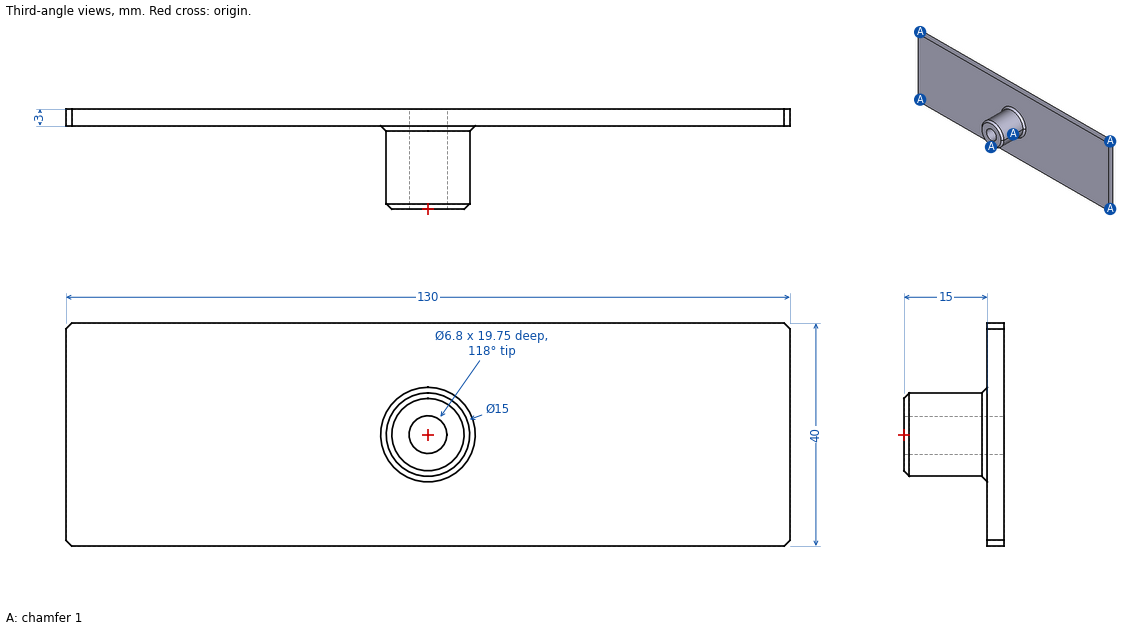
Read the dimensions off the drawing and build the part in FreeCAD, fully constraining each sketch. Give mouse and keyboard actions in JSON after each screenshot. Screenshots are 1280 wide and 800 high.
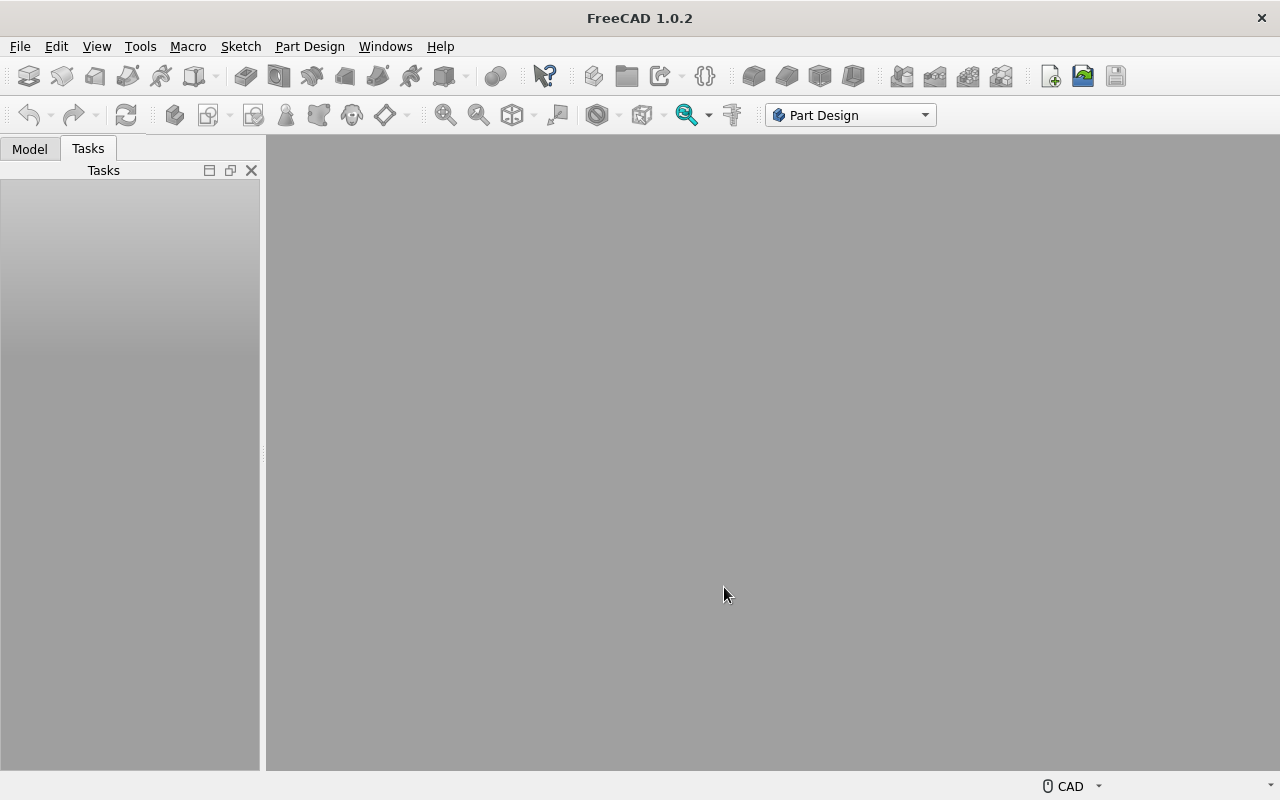
{"action": "left_click", "coordinate": [1050, 76]}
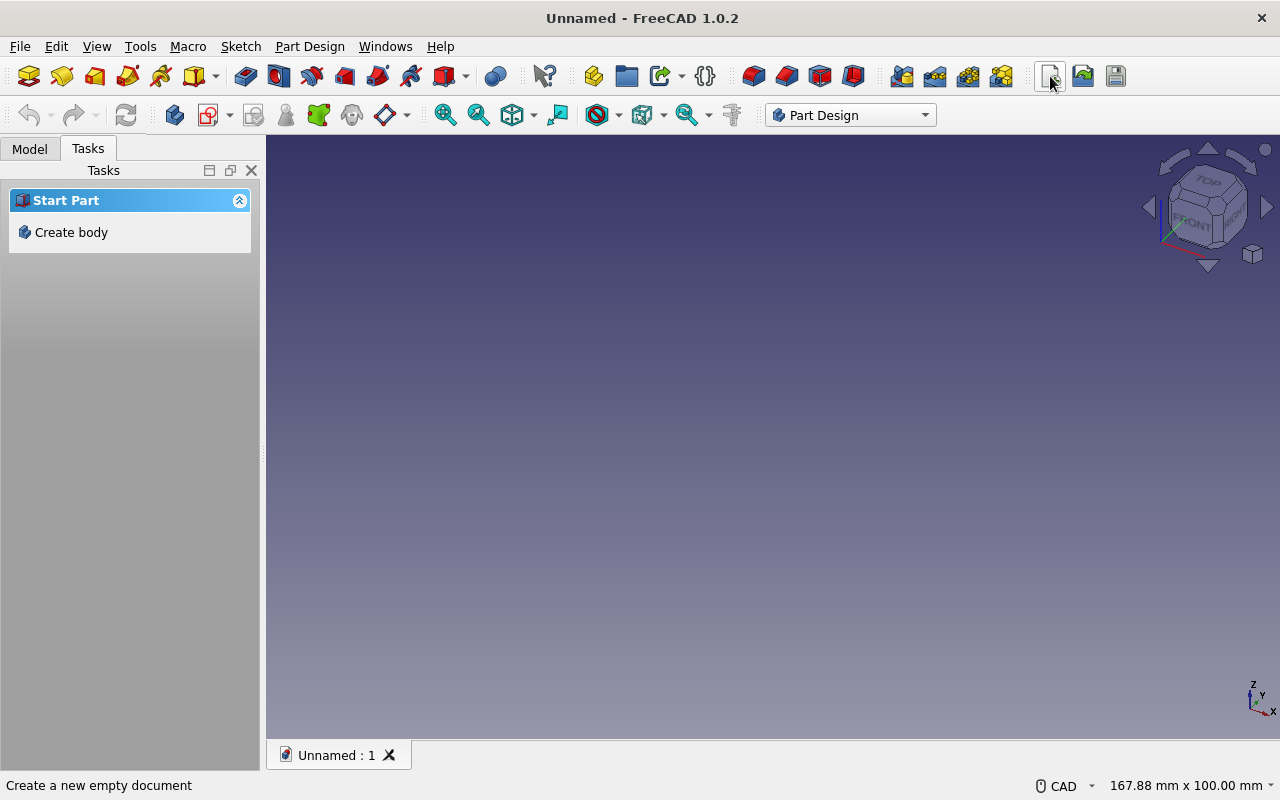
{"action": "left_click", "coordinate": [208, 116]}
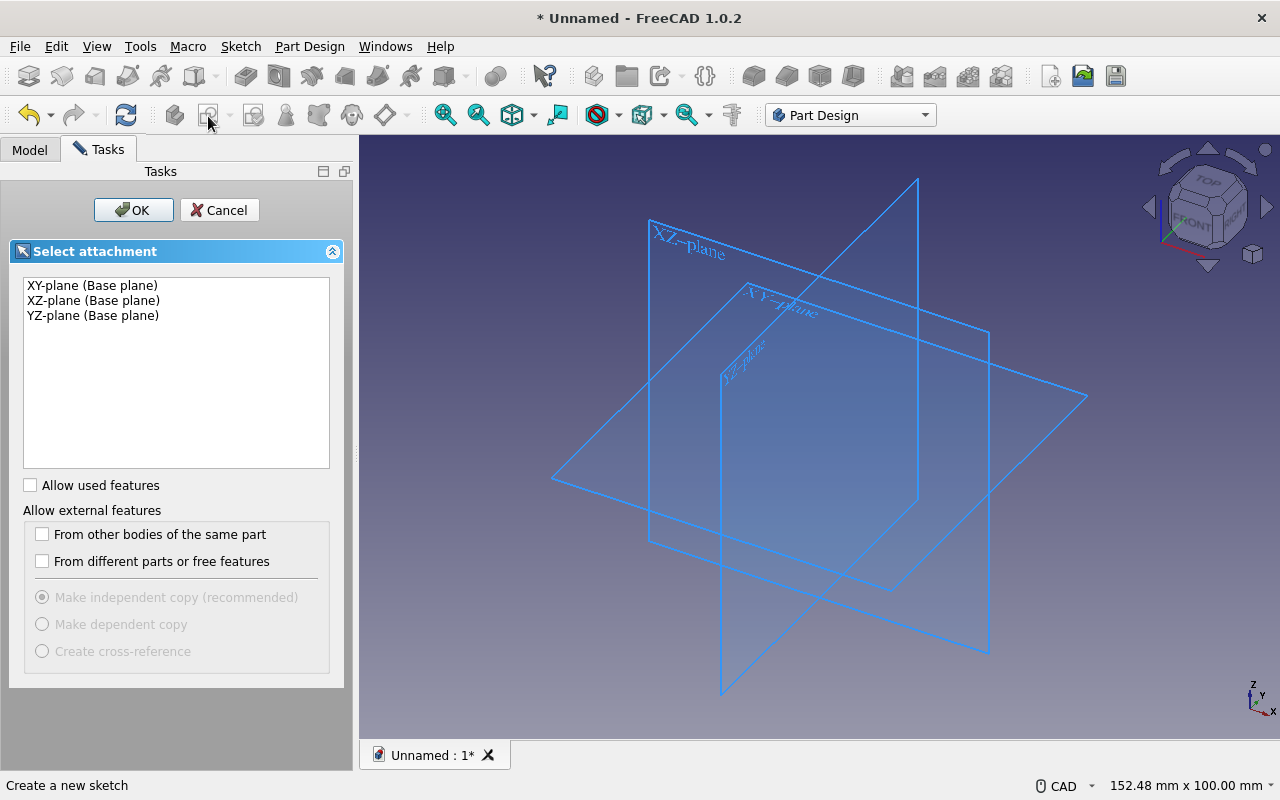
{"action": "left_click", "coordinate": [84, 300]}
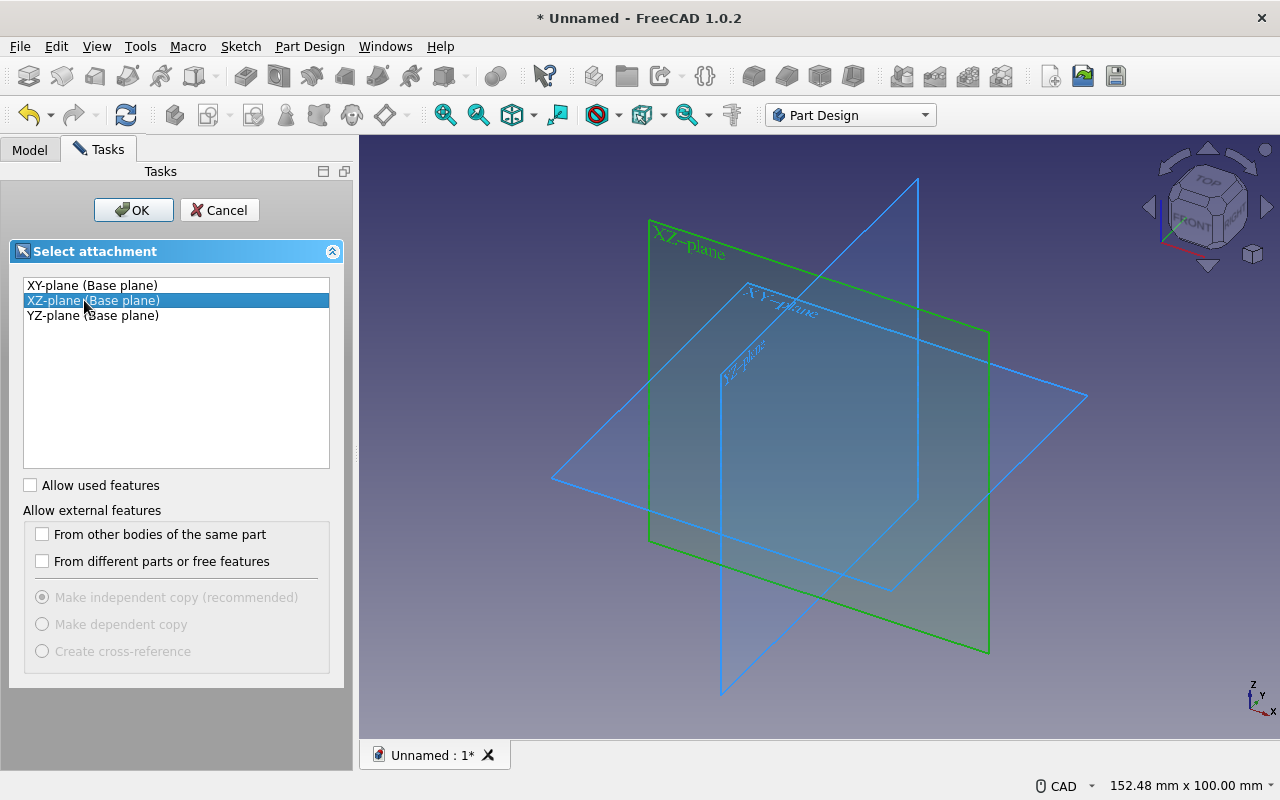
{"action": "left_click", "coordinate": [134, 210]}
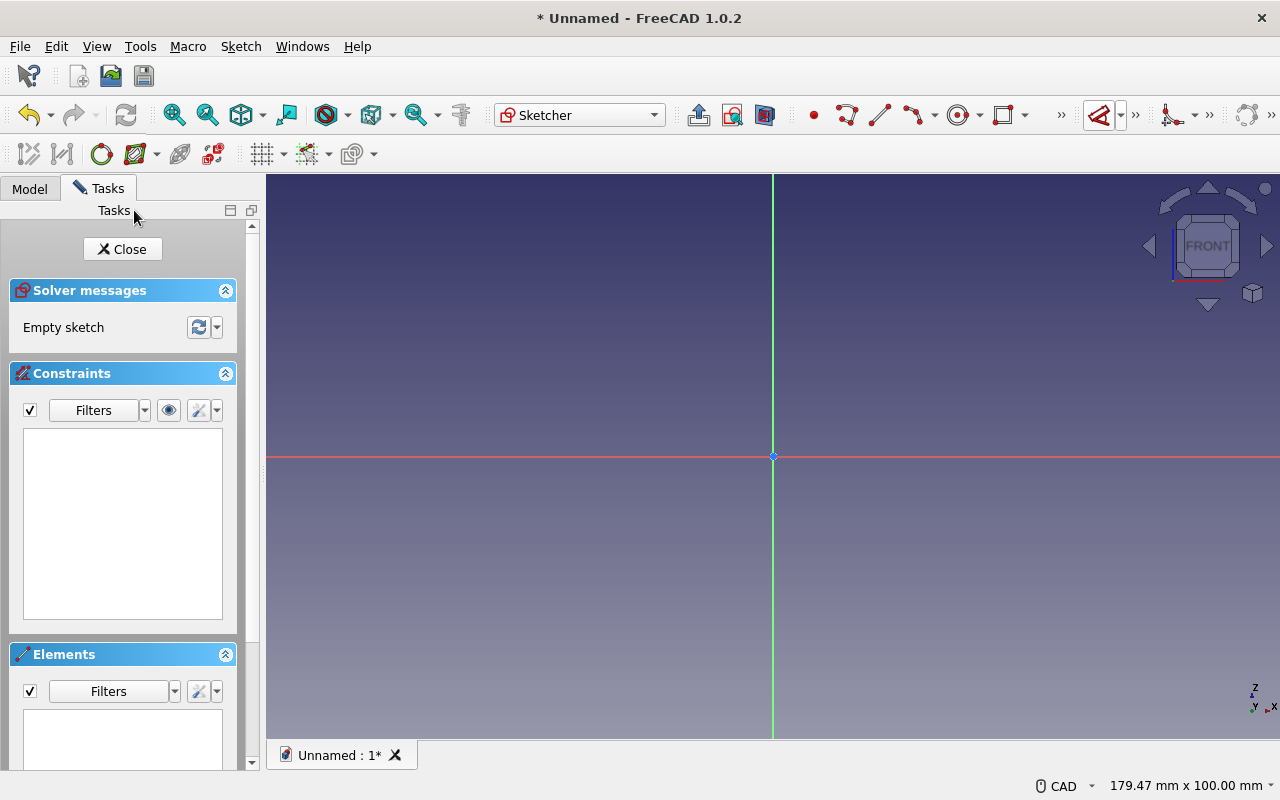
{"action": "scroll", "coordinate": [795, 456], "scroll_direction": "up", "scroll_amount": 7}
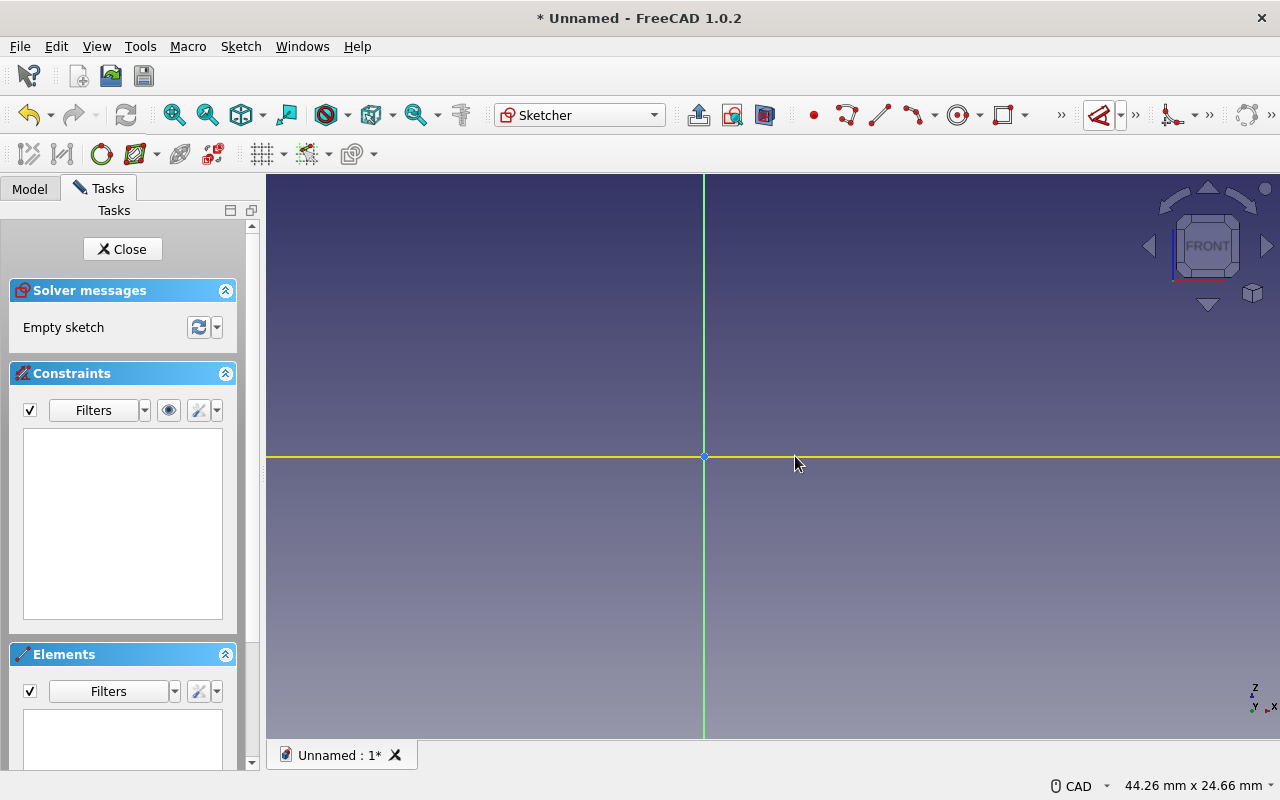
{"action": "left_click", "coordinate": [958, 116]}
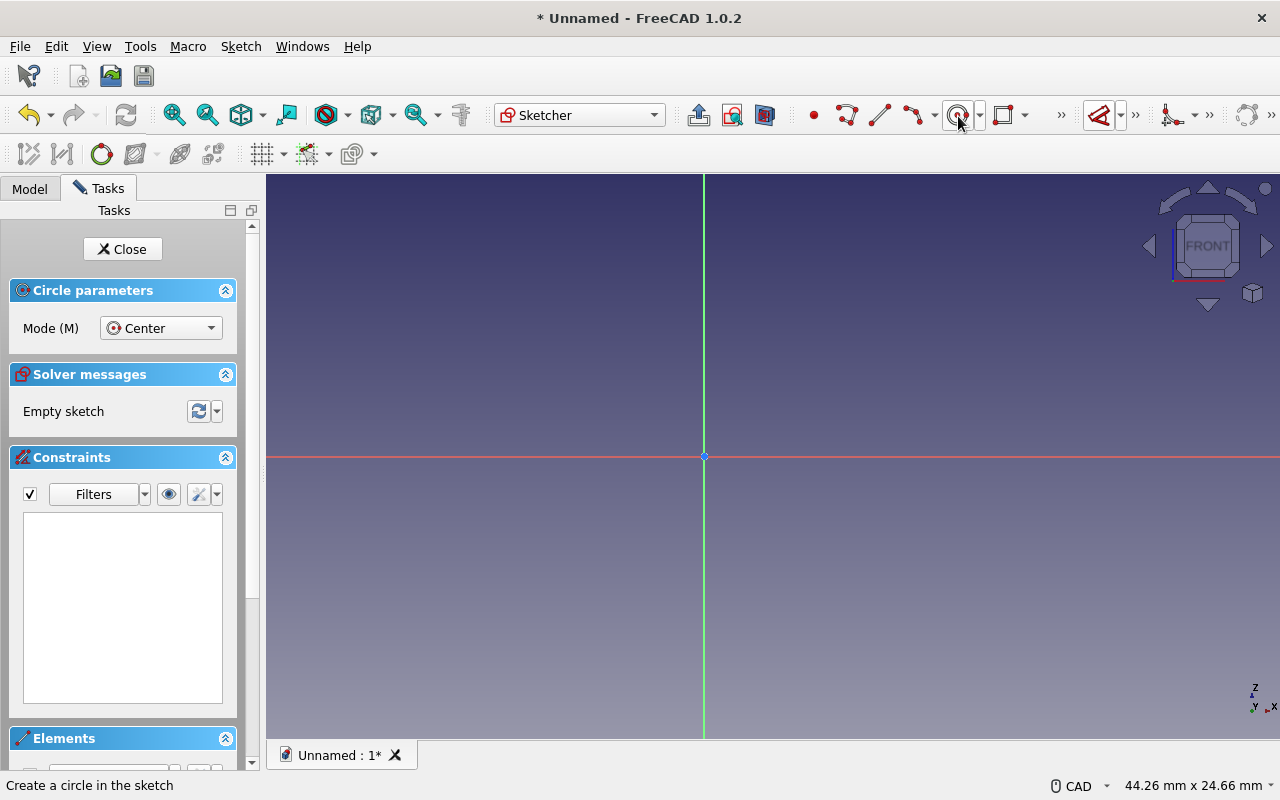
{"action": "left_click", "coordinate": [704, 456]}
{"action": "mouse_move", "coordinate": [826, 335]}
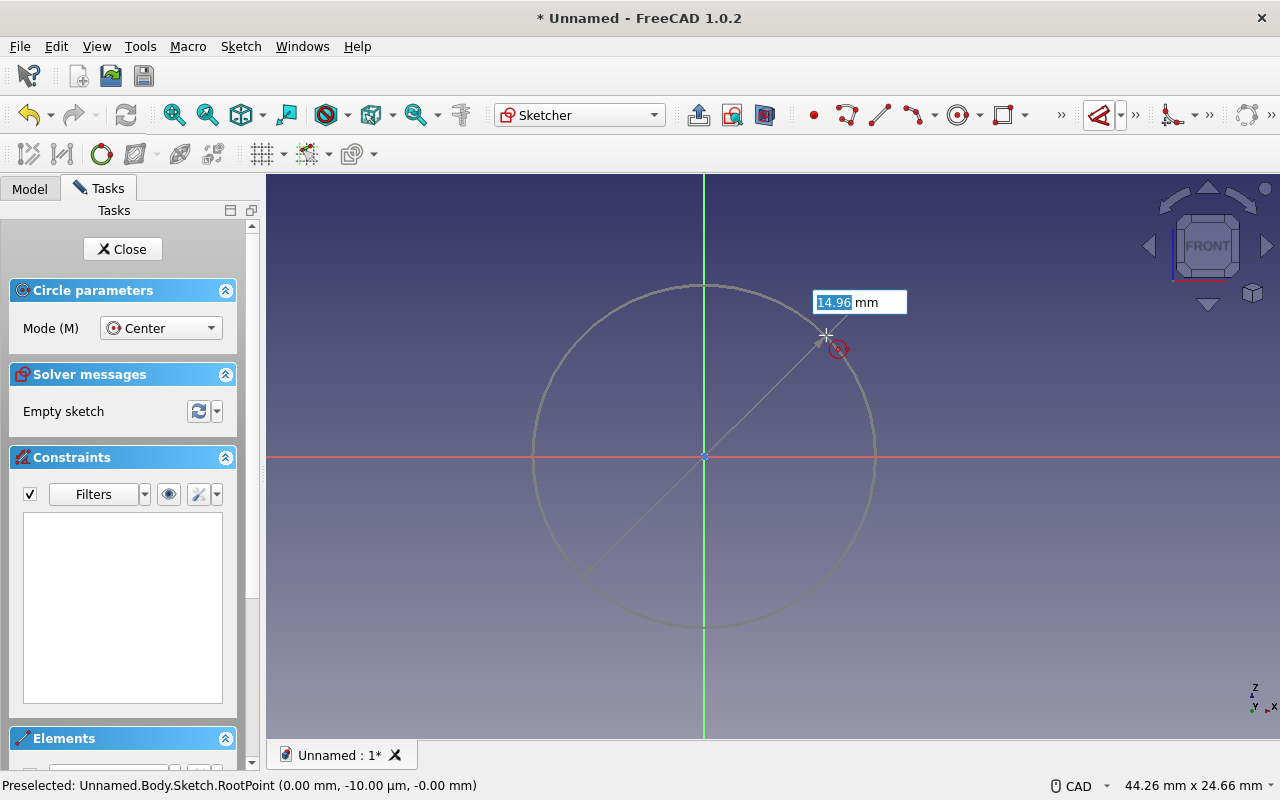
{"action": "type", "text": "15"}
{"action": "key", "text": "Return"}
{"action": "key", "text": "Escape"}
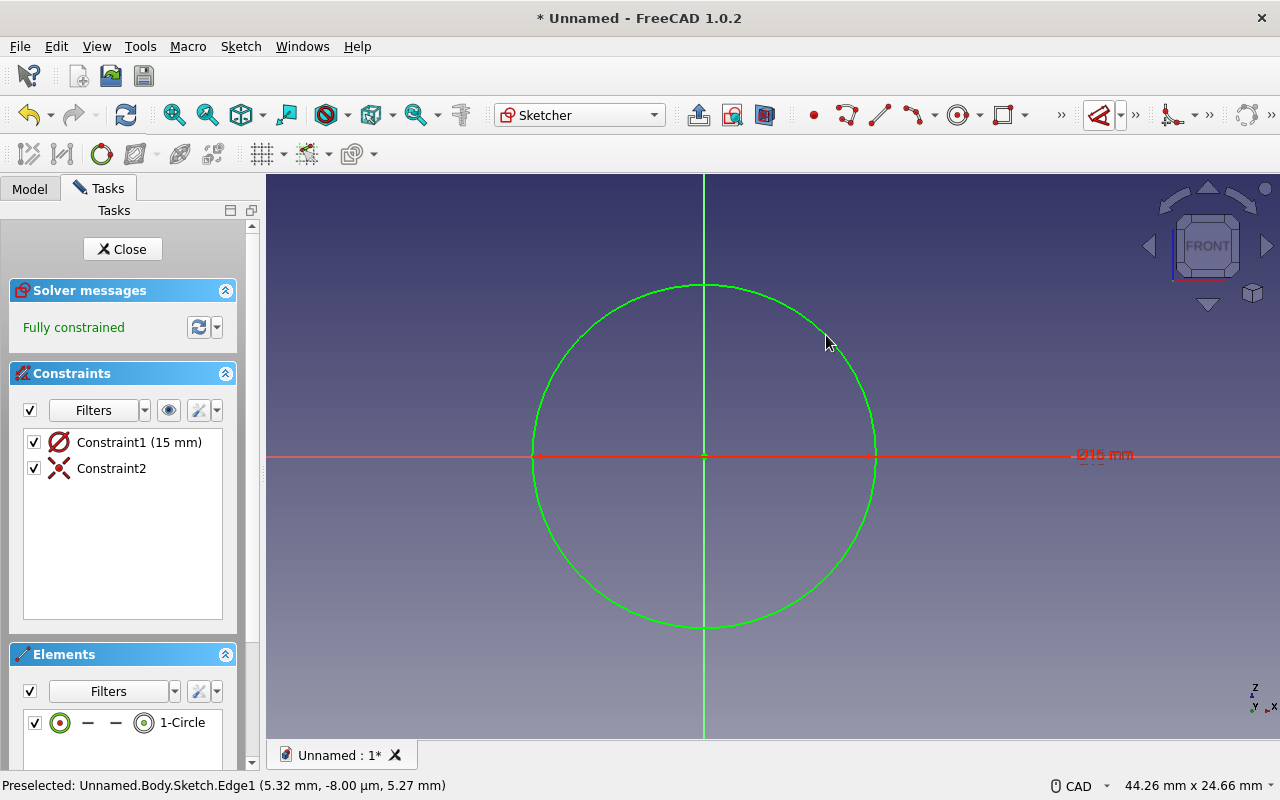
{"action": "left_click", "coordinate": [123, 249]}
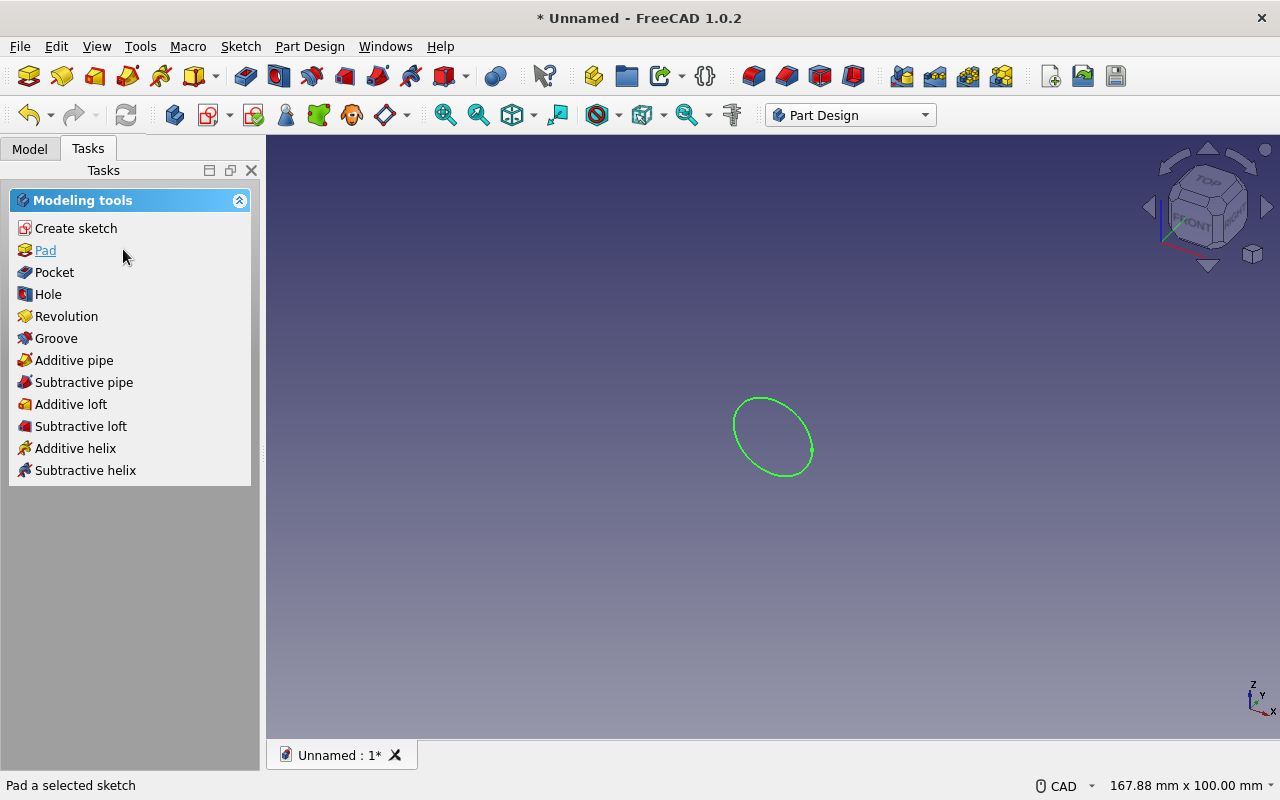
{"action": "left_click", "coordinate": [29, 76]}